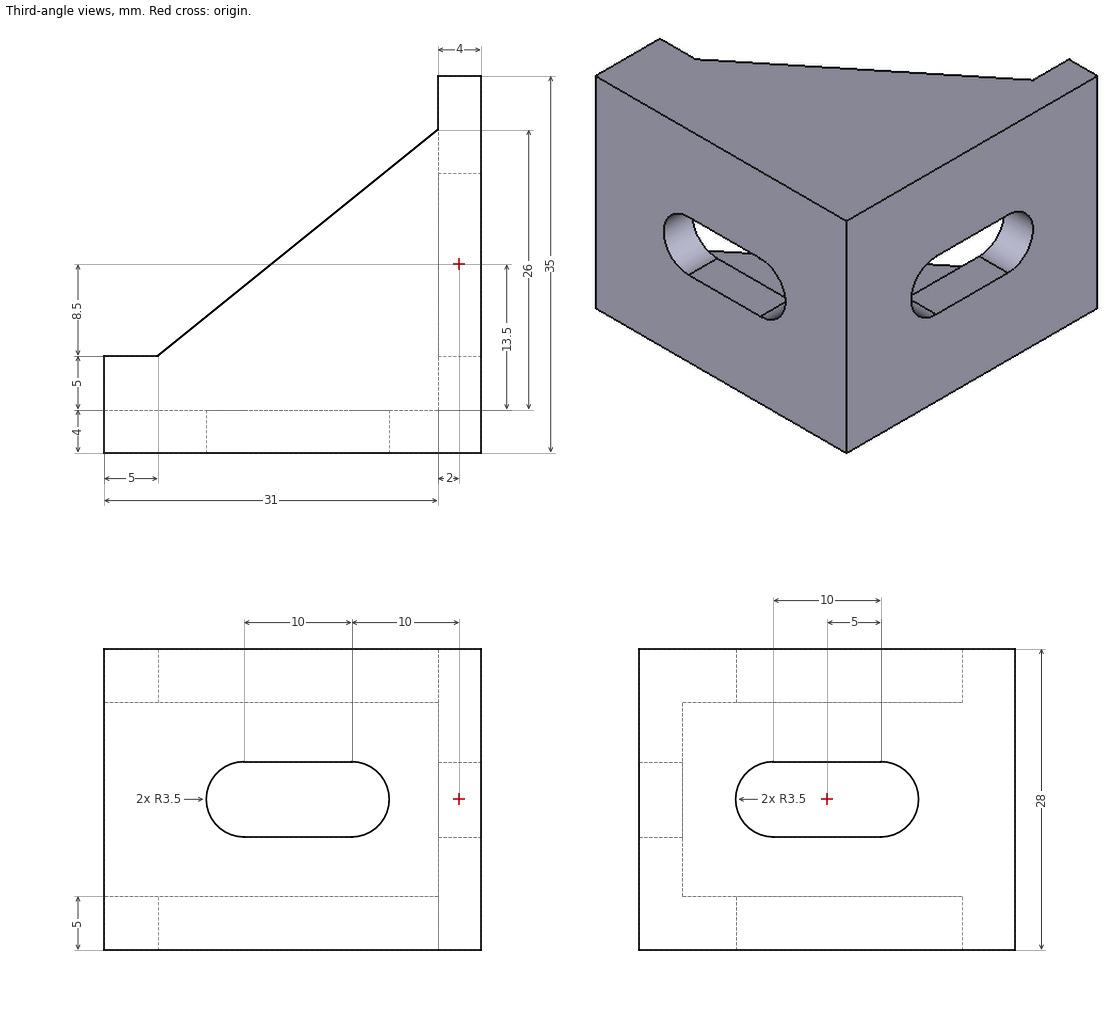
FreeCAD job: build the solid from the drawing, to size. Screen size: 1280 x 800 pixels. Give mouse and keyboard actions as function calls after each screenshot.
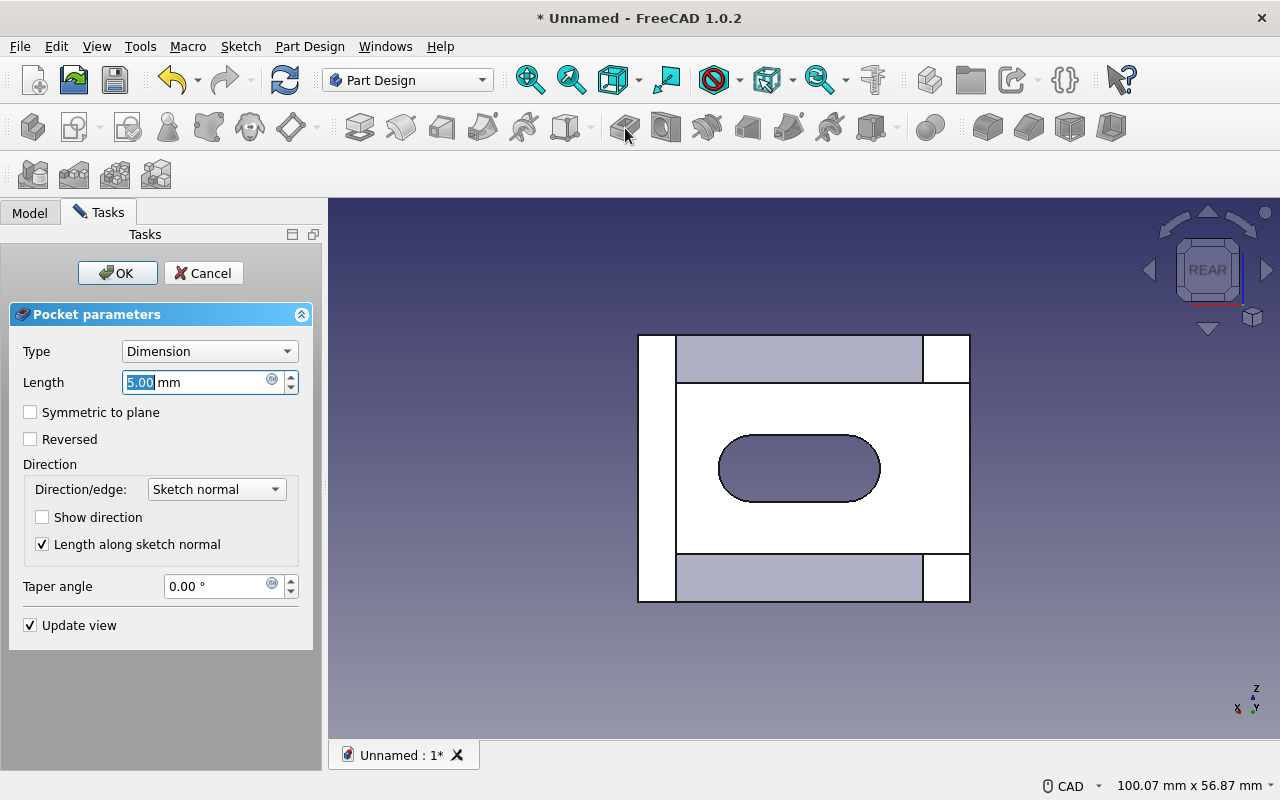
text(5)
key(Tab)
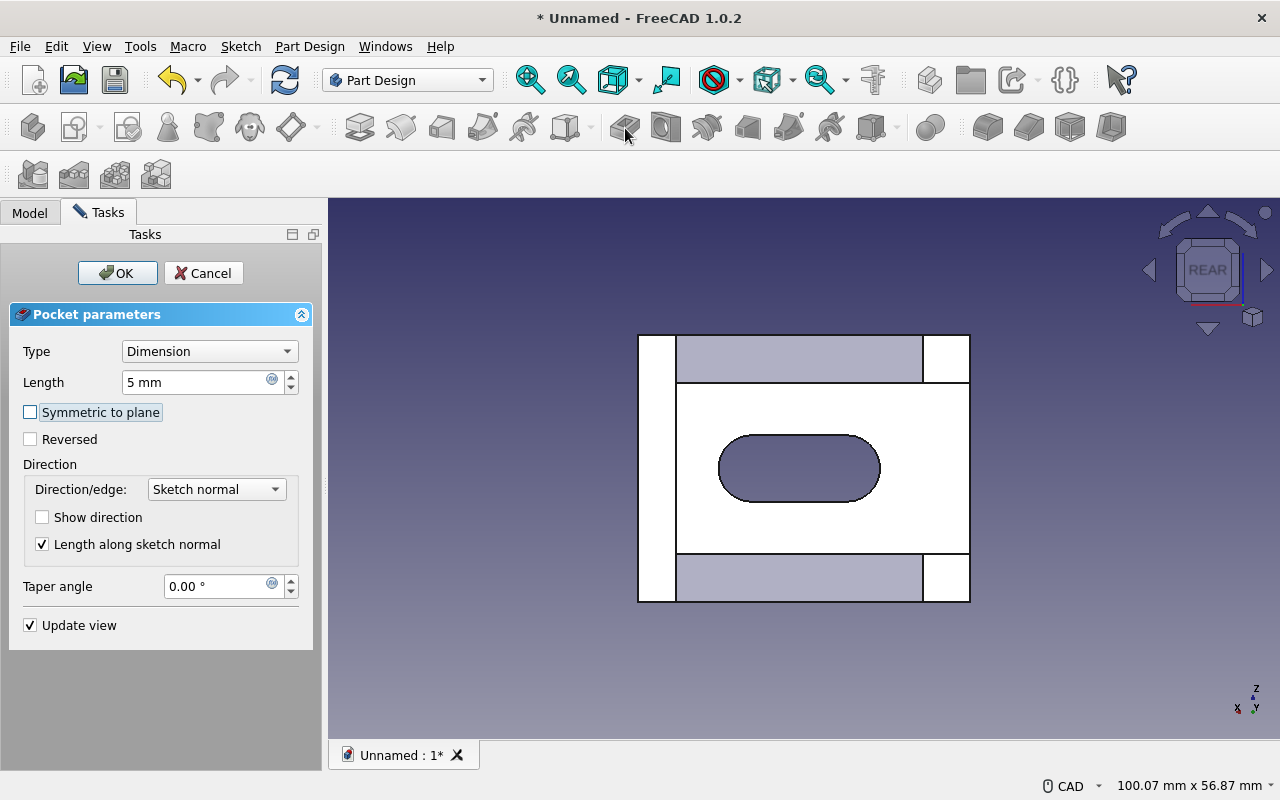
click(118, 273)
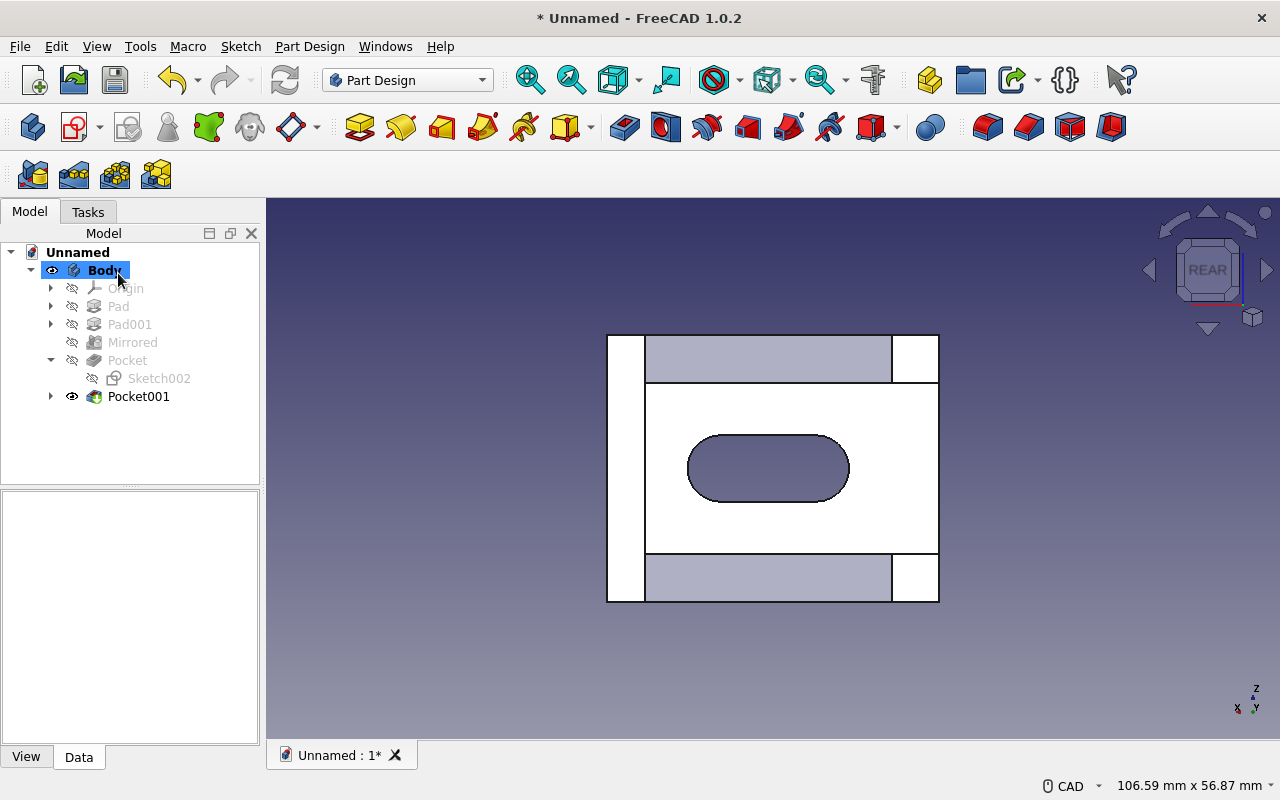
key(0)